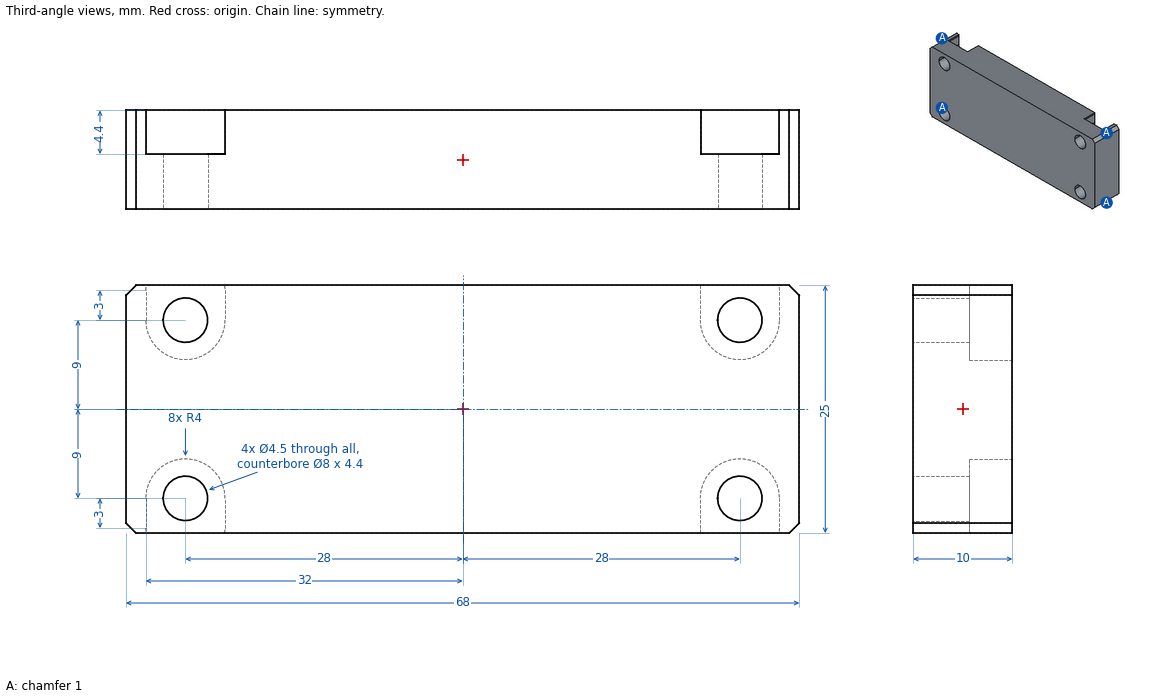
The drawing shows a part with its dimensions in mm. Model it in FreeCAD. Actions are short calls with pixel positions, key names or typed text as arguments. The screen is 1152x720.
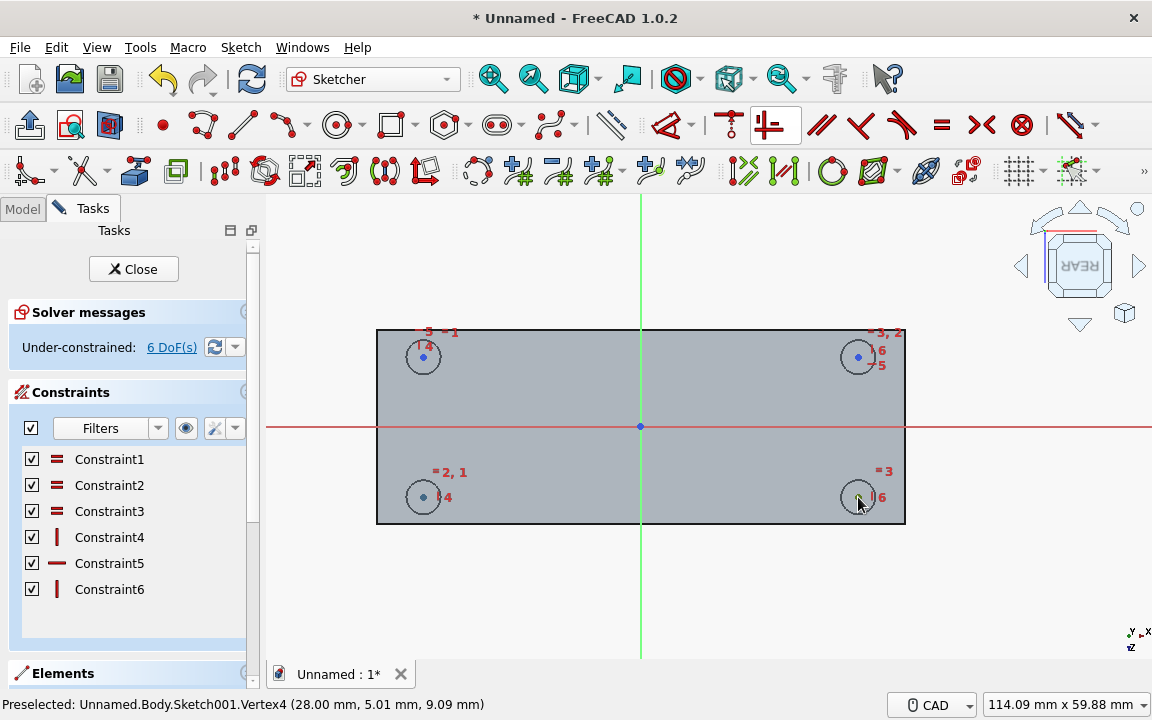
click(796, 126)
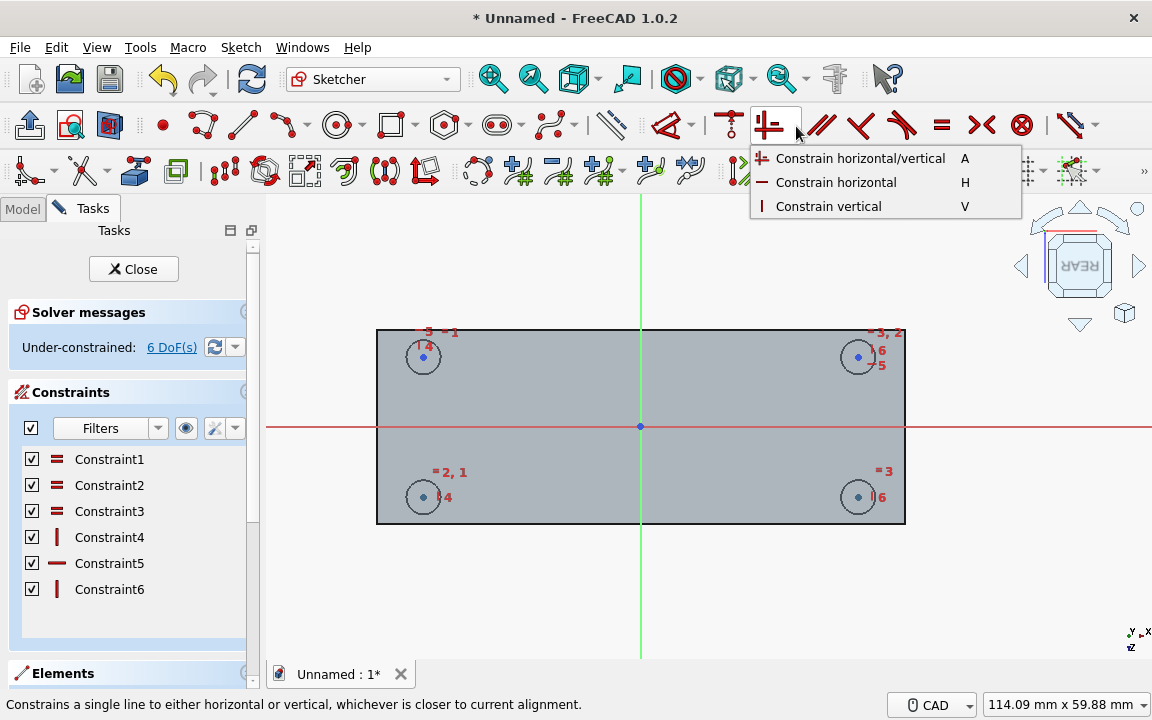
click(886, 182)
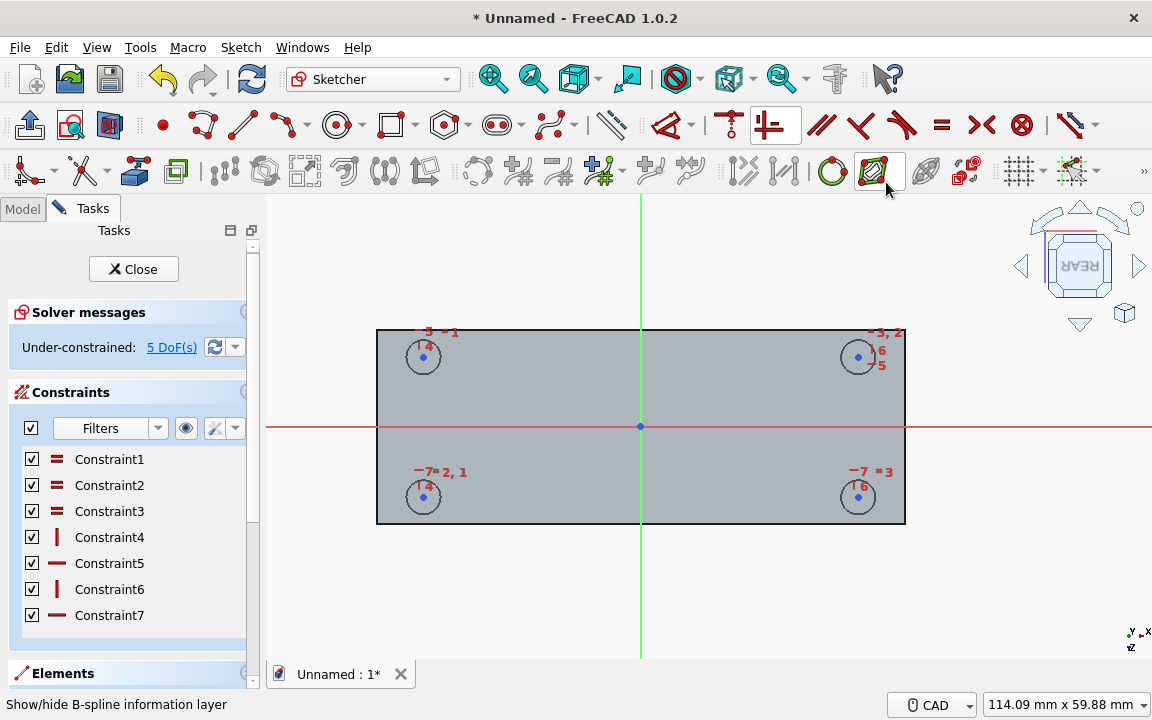
click(666, 126)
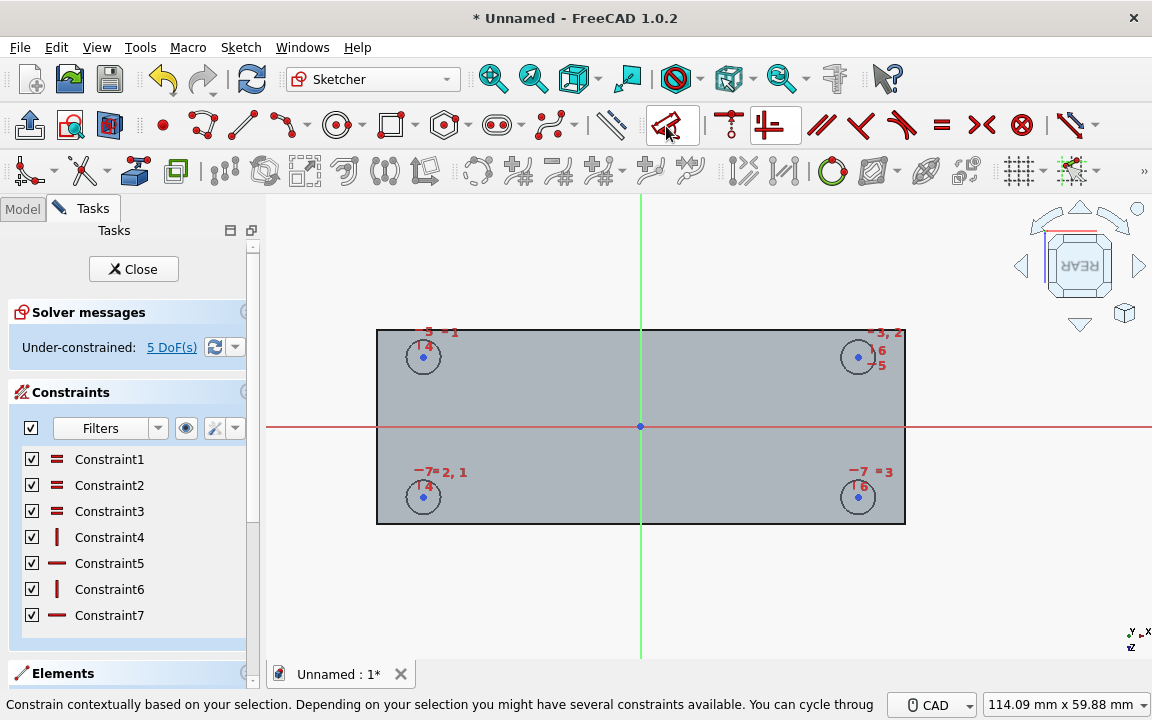
click(436, 345)
click(459, 323)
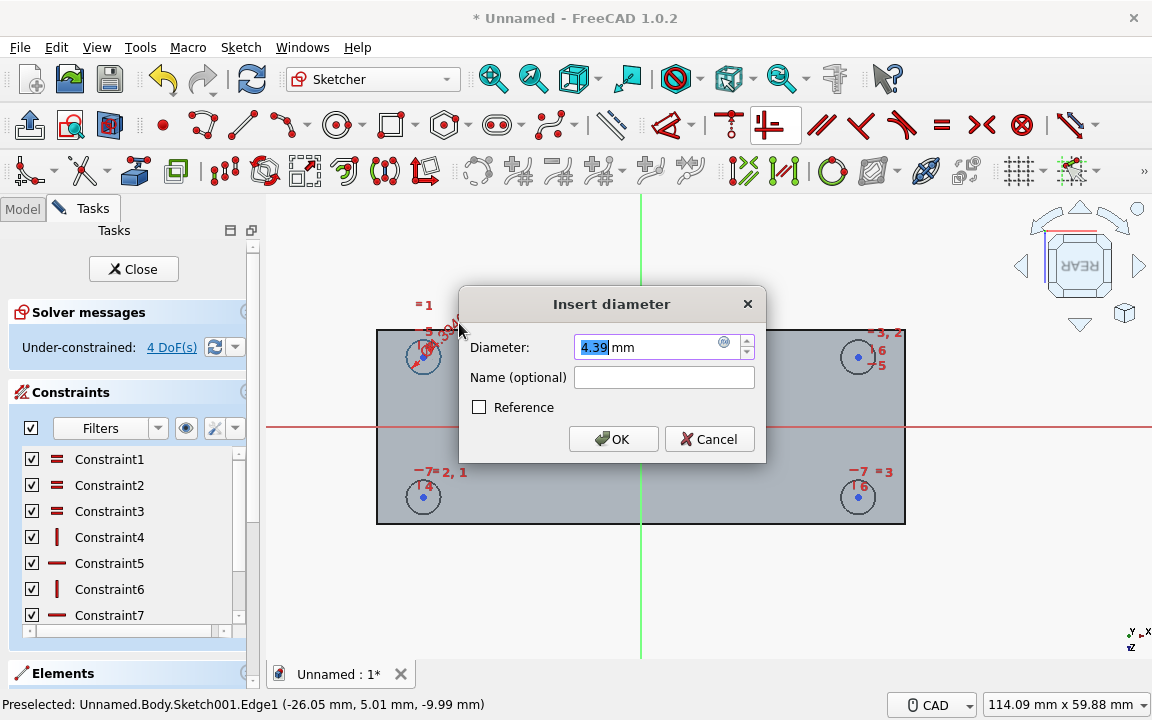
text(4.5)
key(Return)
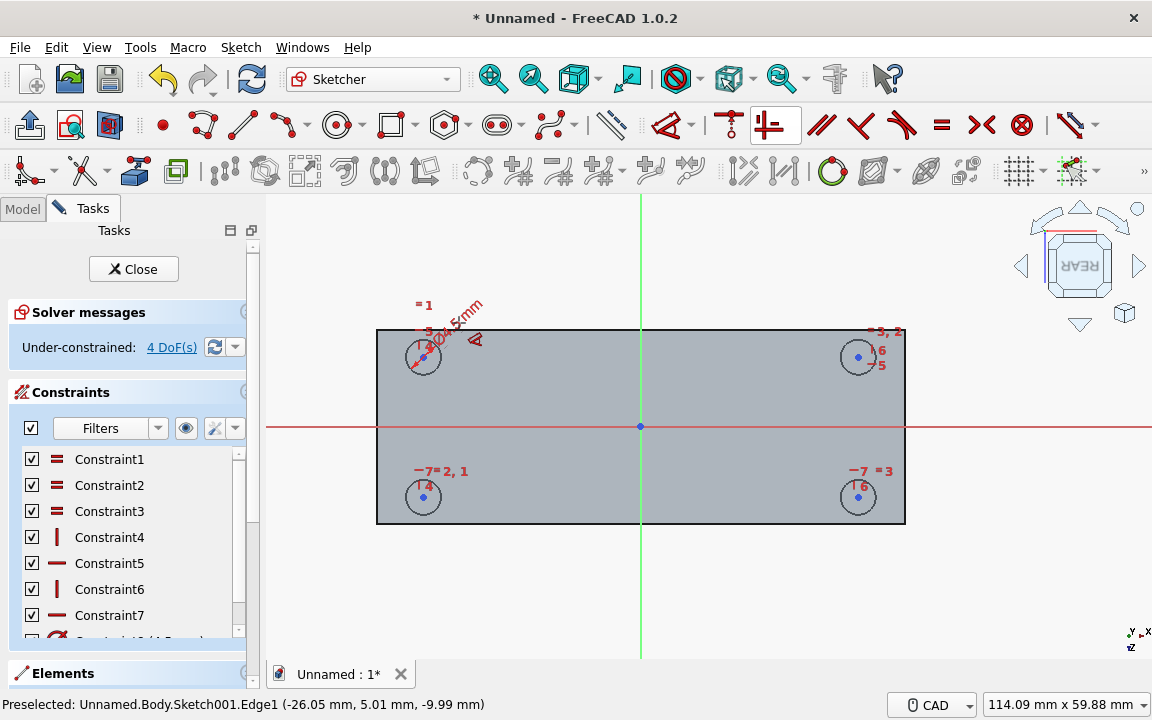
click(424, 357)
click(390, 392)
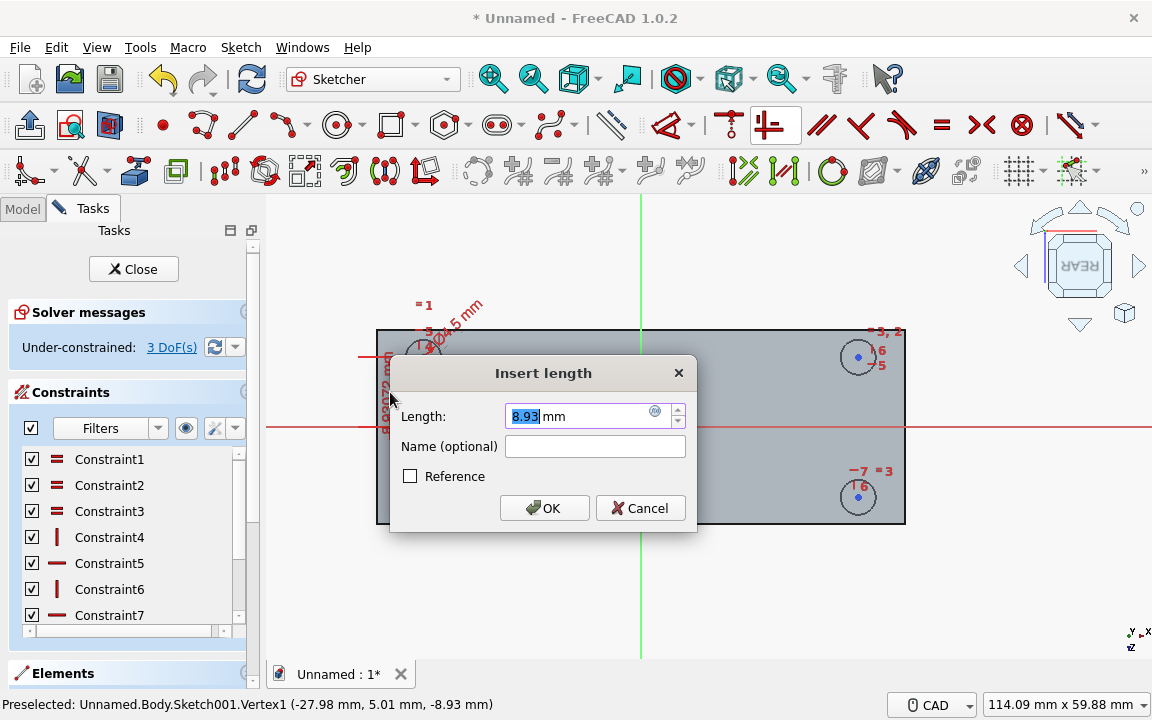
text(9)
key(Return)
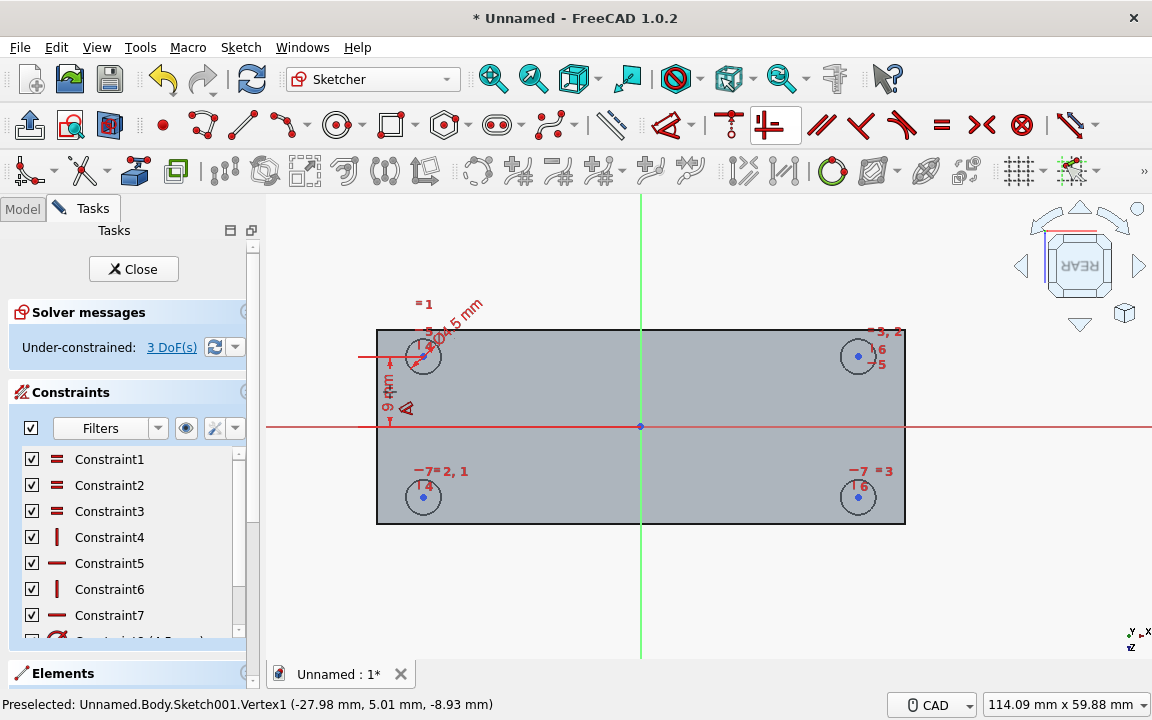
click(424, 497)
click(390, 462)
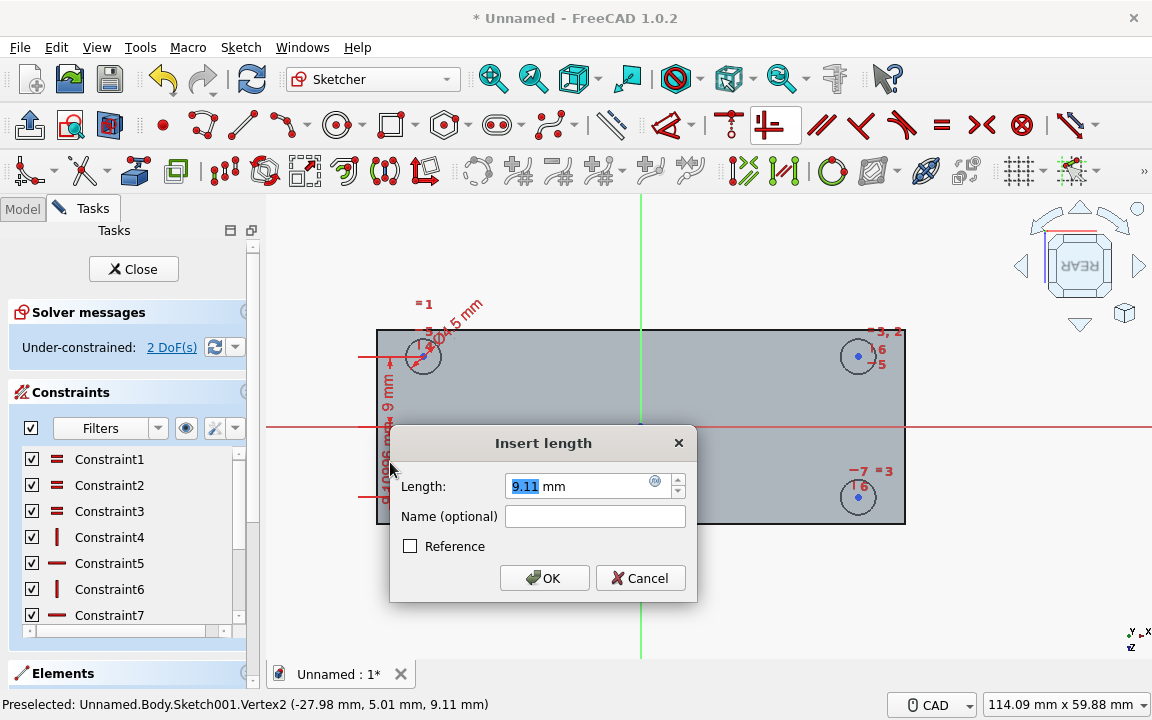
text(9)
key(Return)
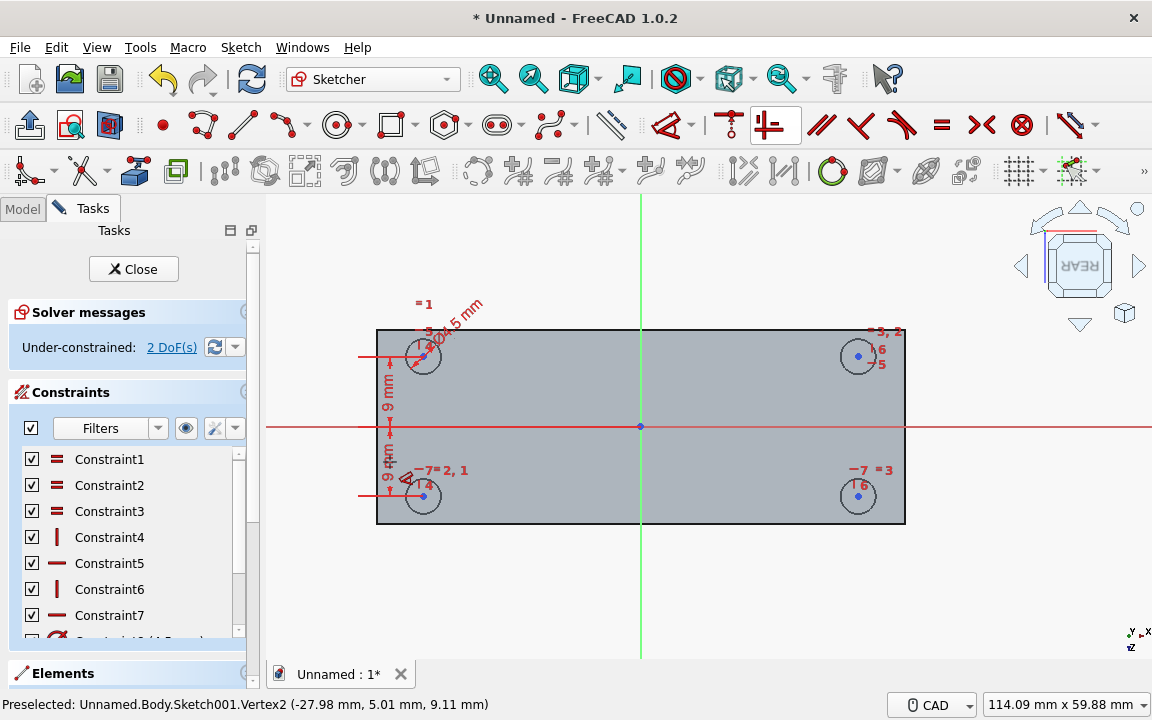
click(424, 357)
click(532, 323)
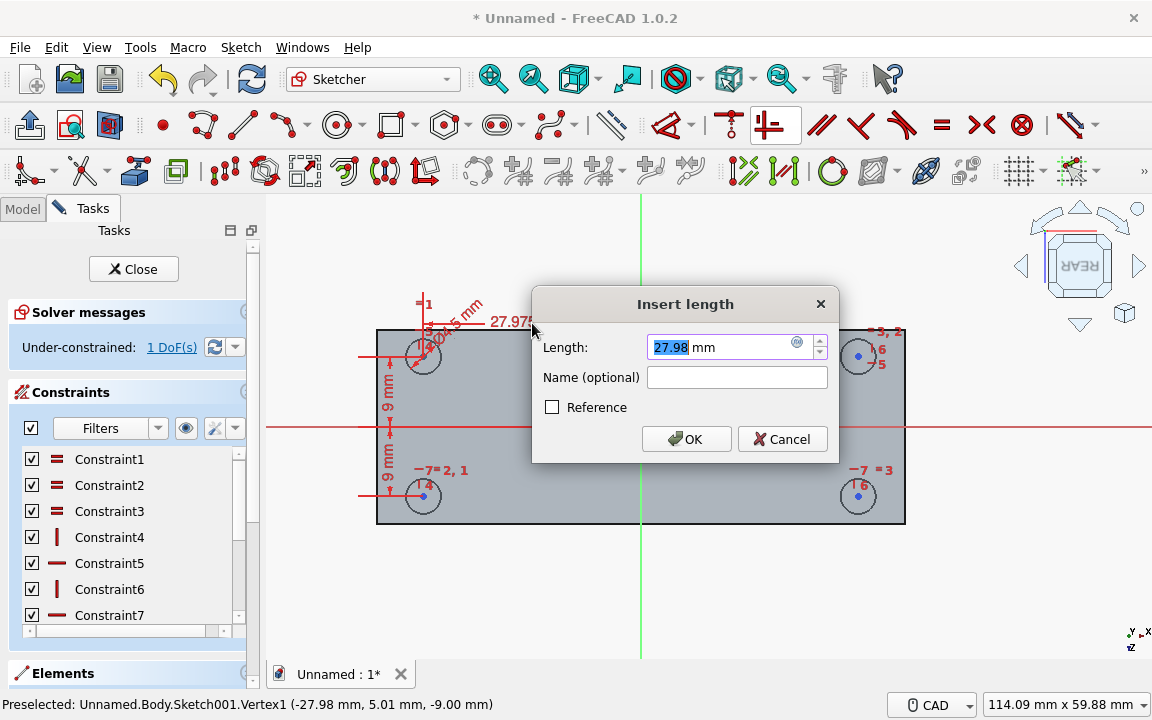
text(28)
key(Return)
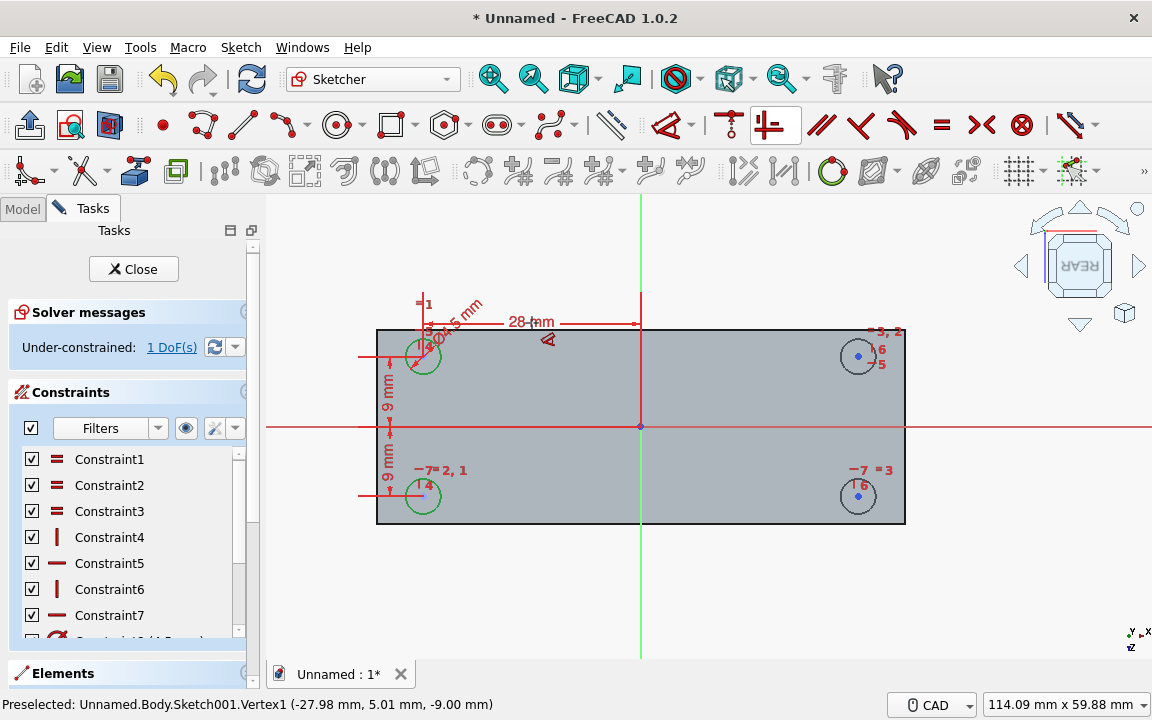
click(858, 357)
click(749, 323)